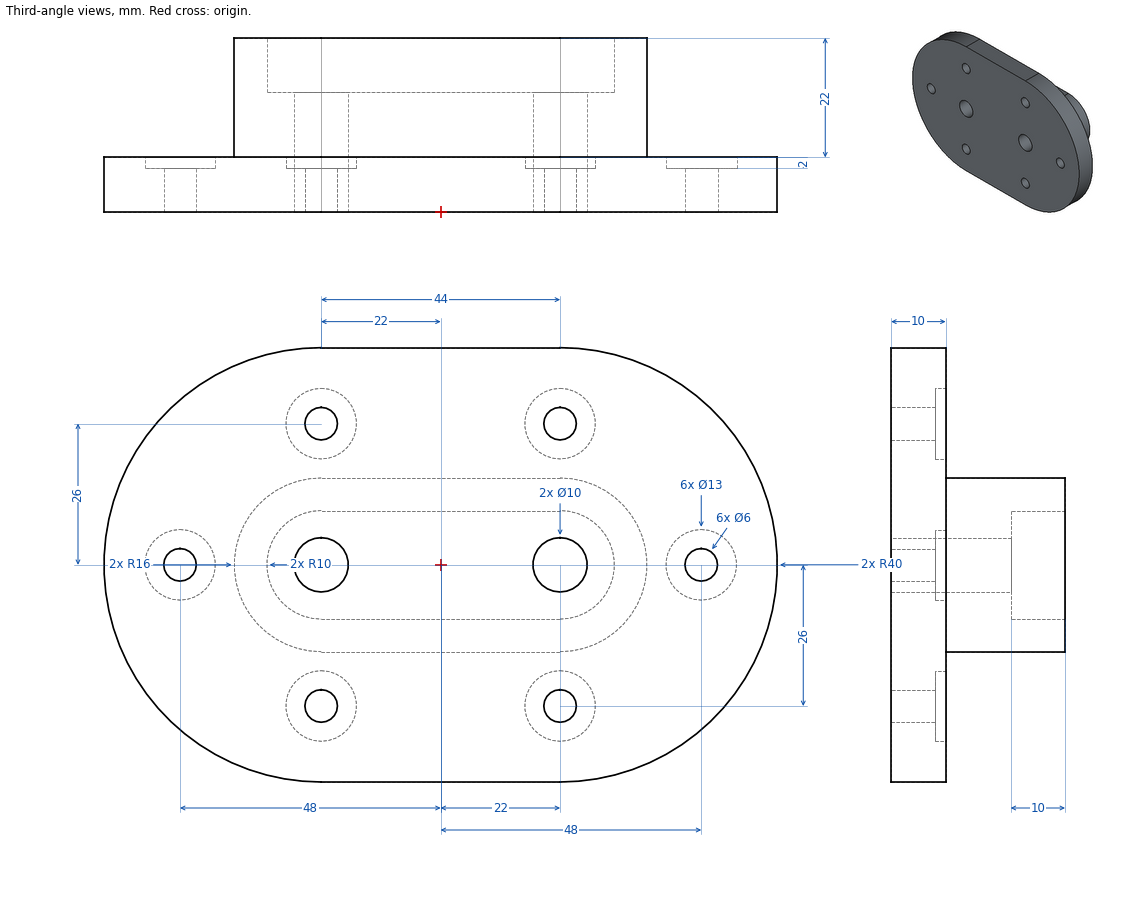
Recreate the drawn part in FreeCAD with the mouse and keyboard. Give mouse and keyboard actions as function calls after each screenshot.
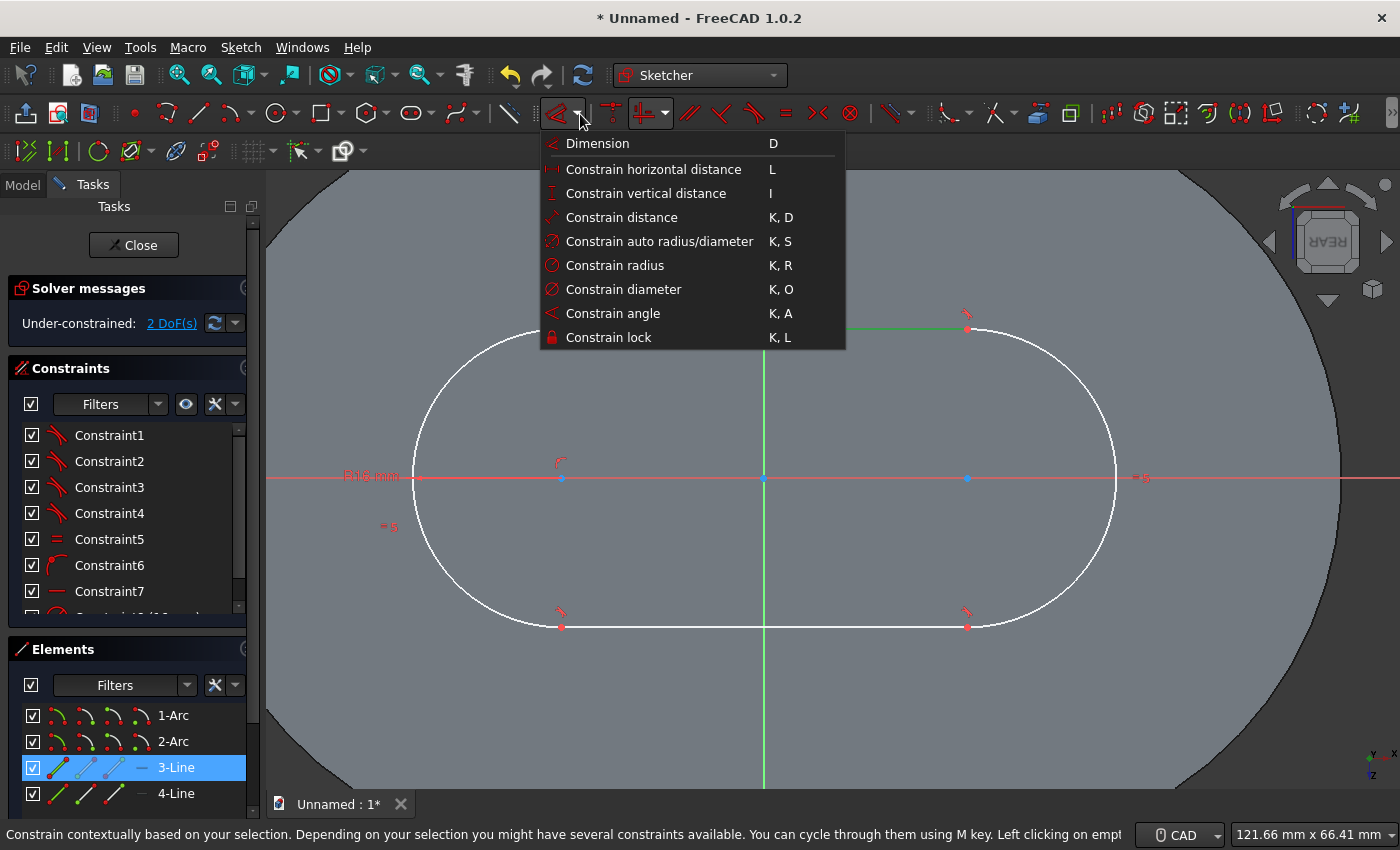
click(693, 169)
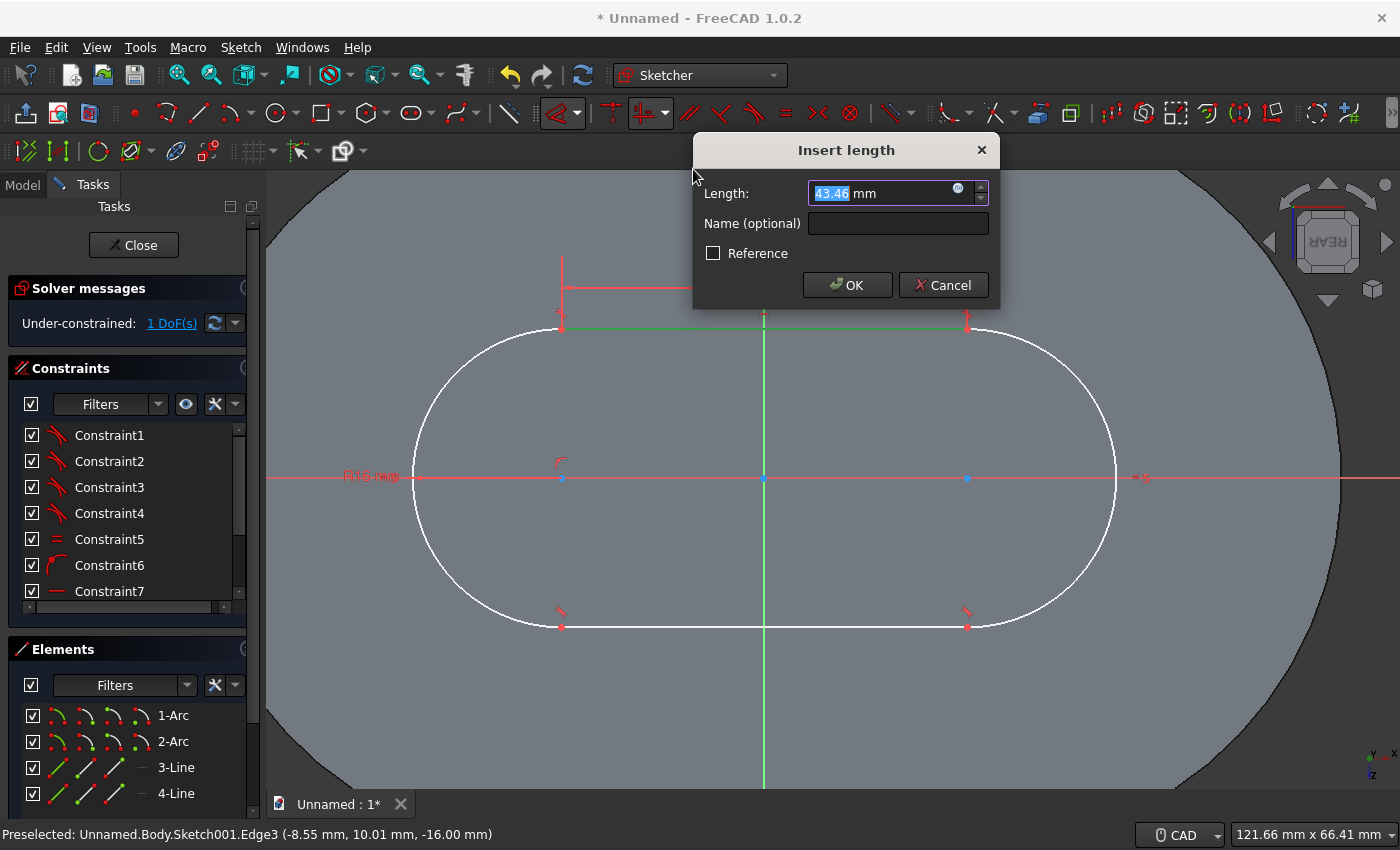
text(44)
key(Return)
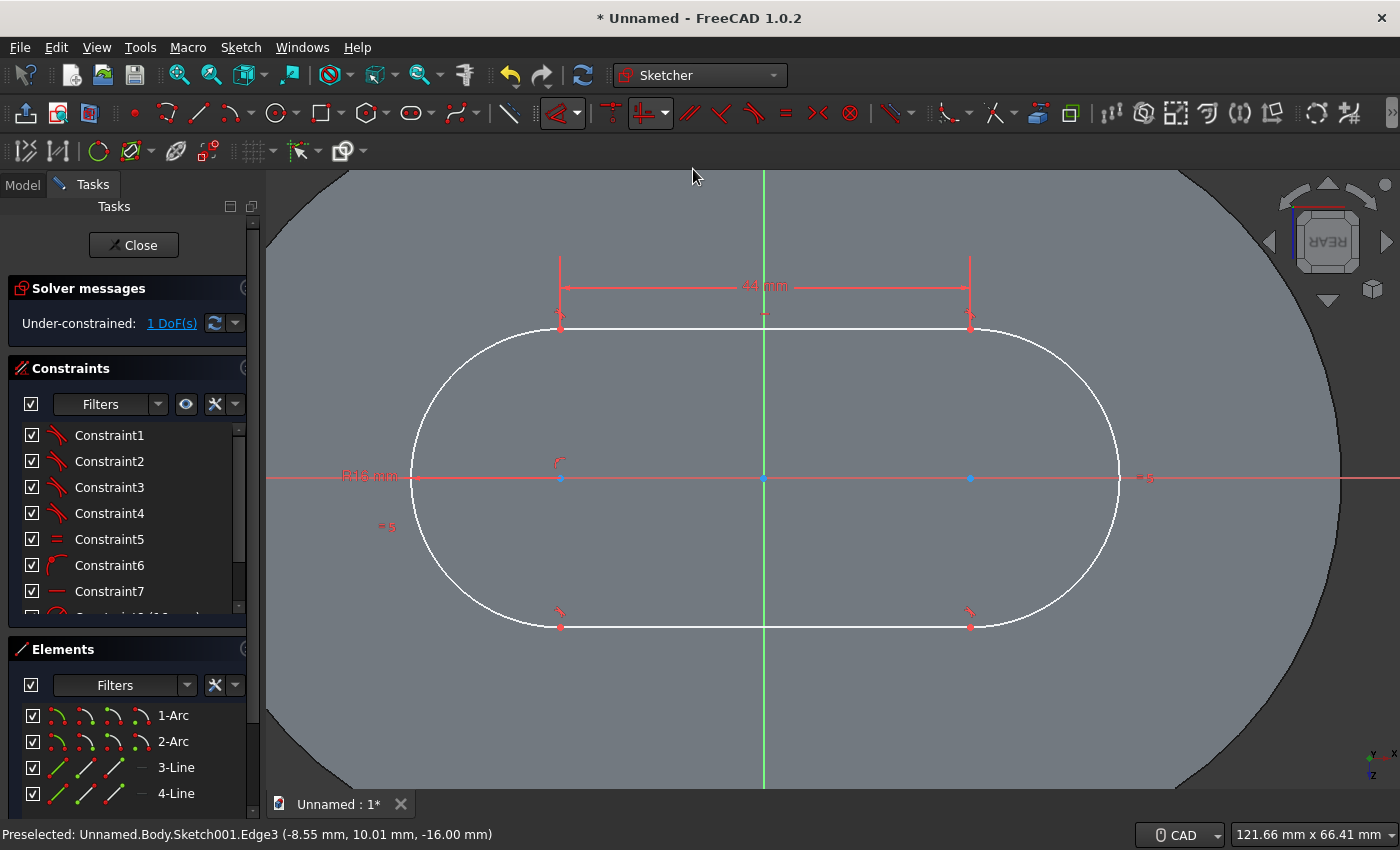
click(560, 329)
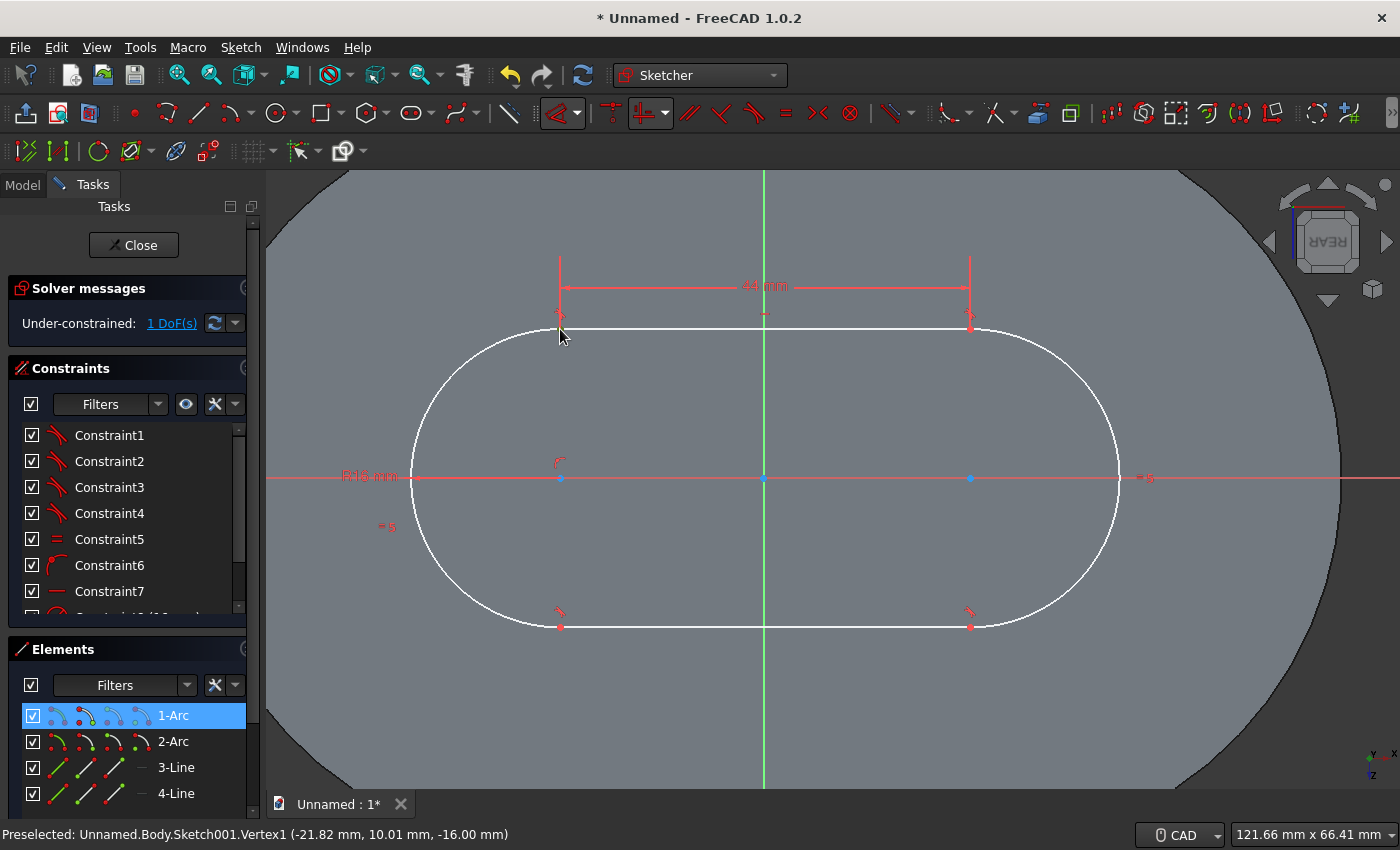
key(l)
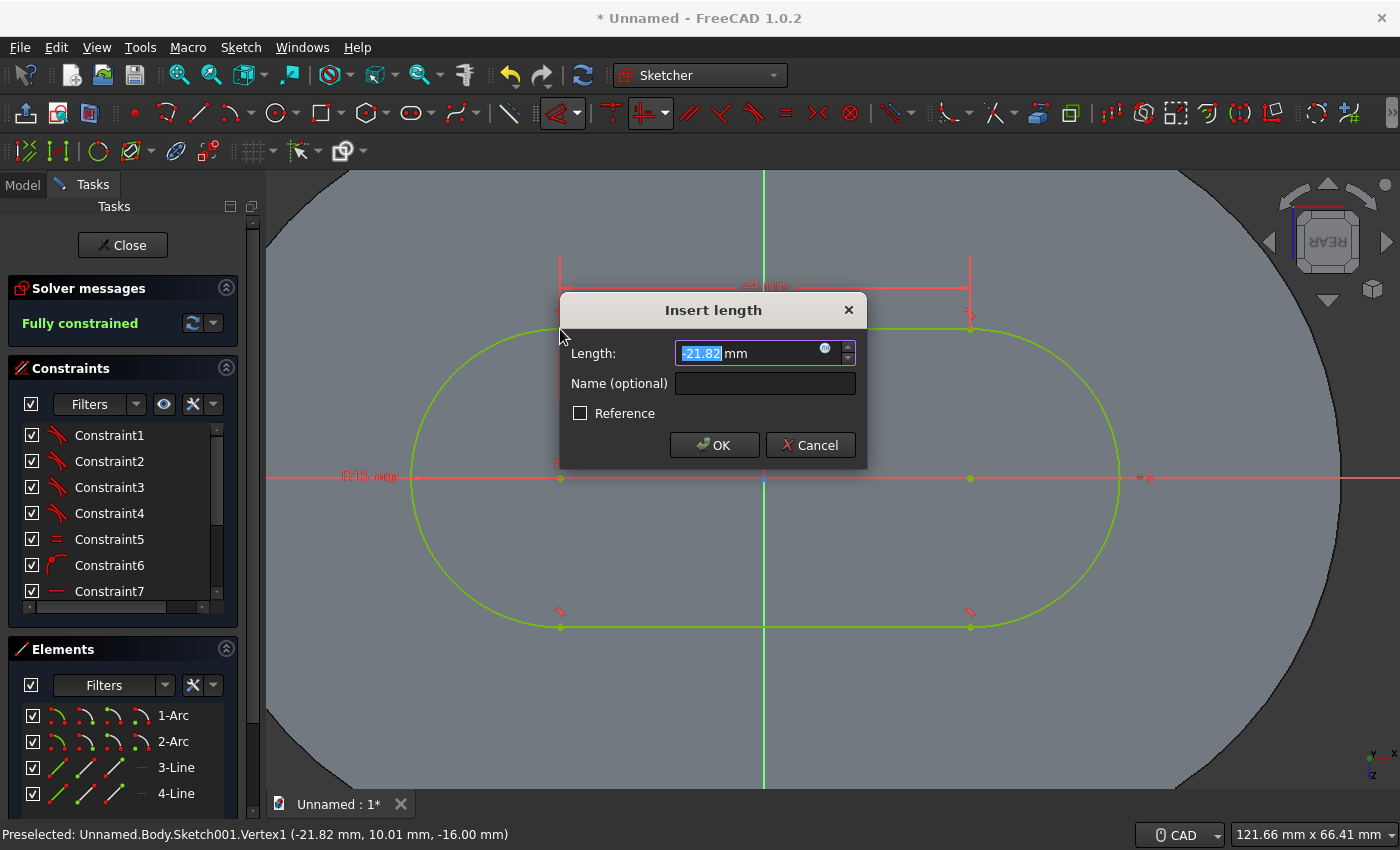
text(-22)
key(Return)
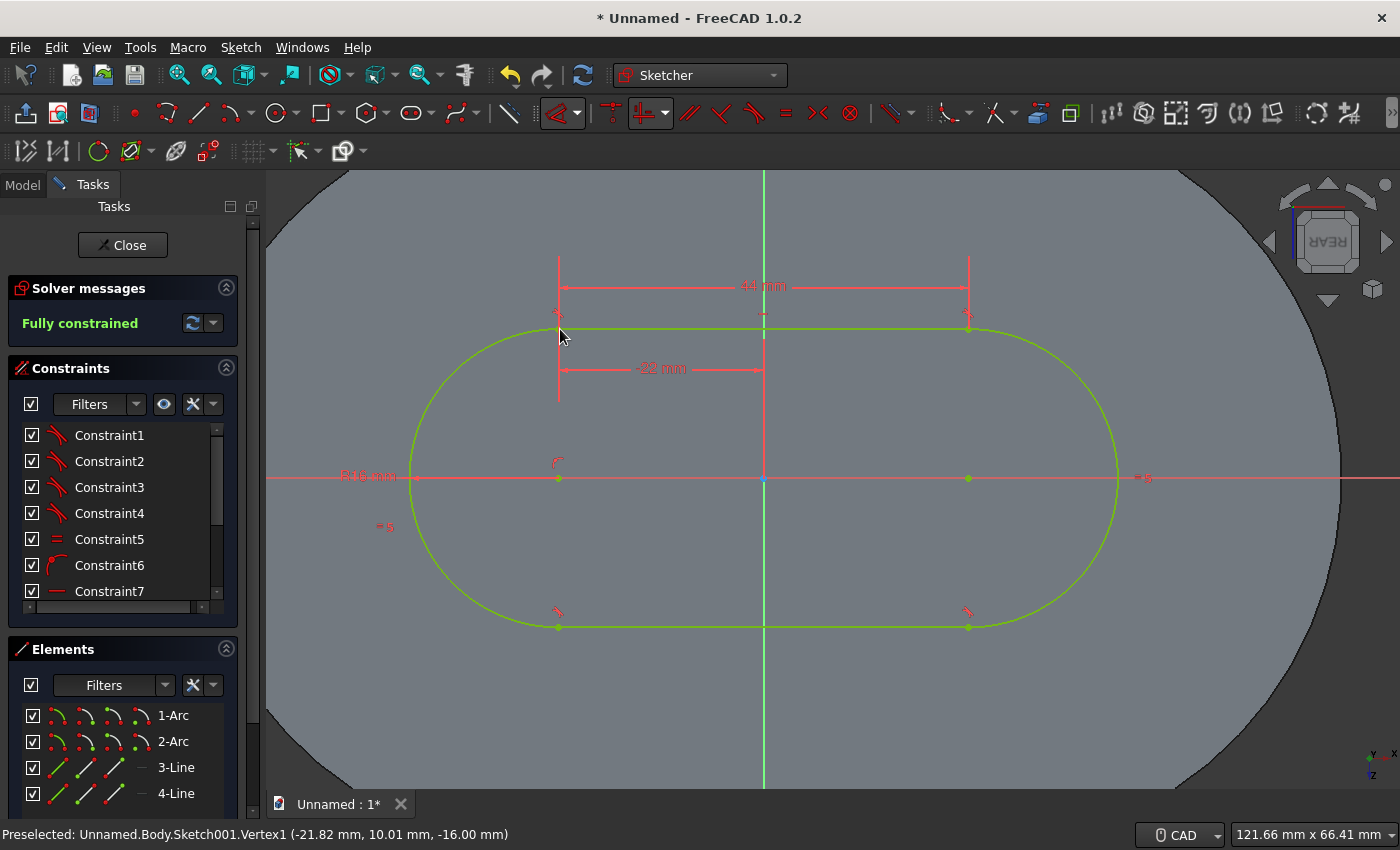
click(123, 245)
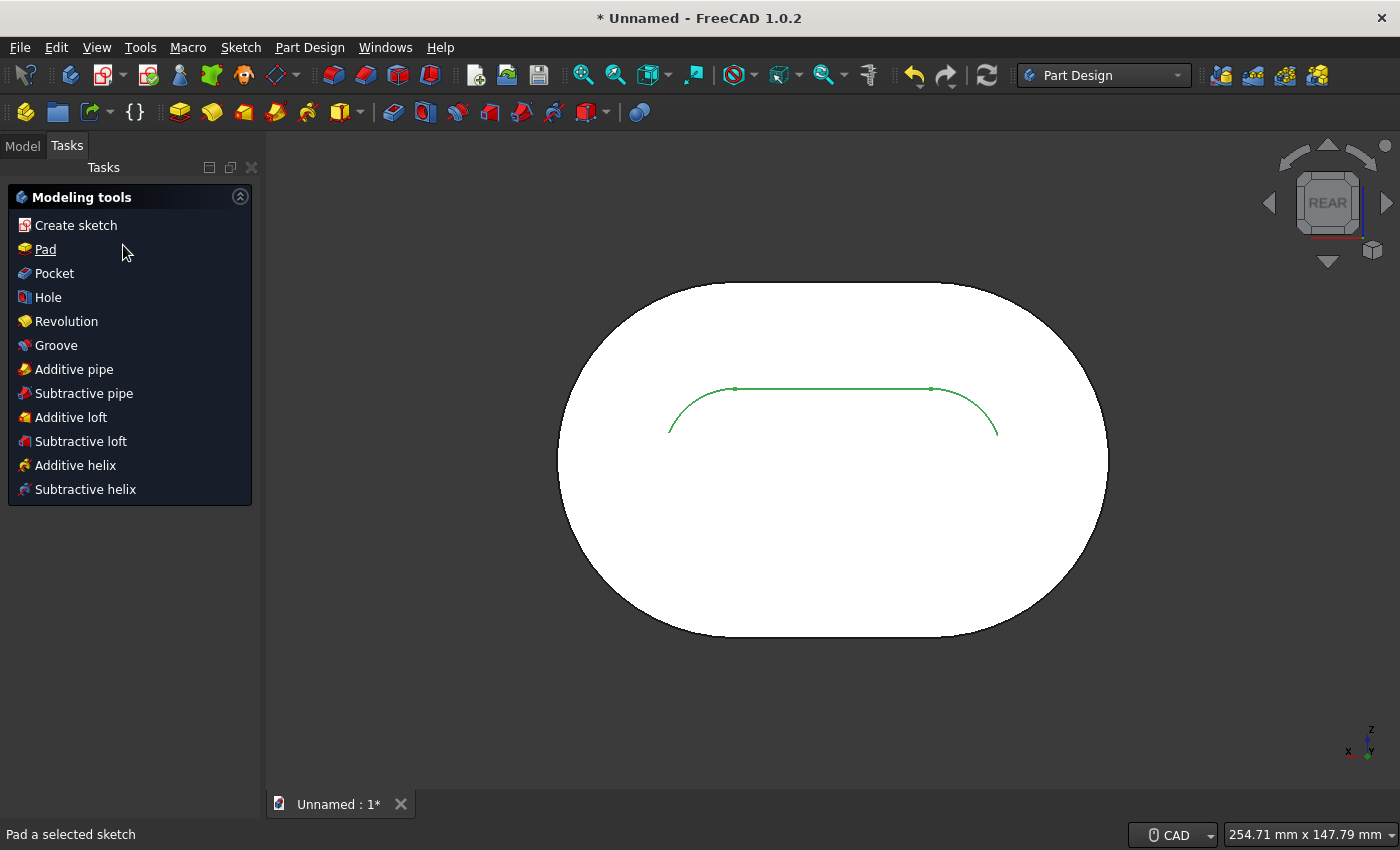
click(180, 112)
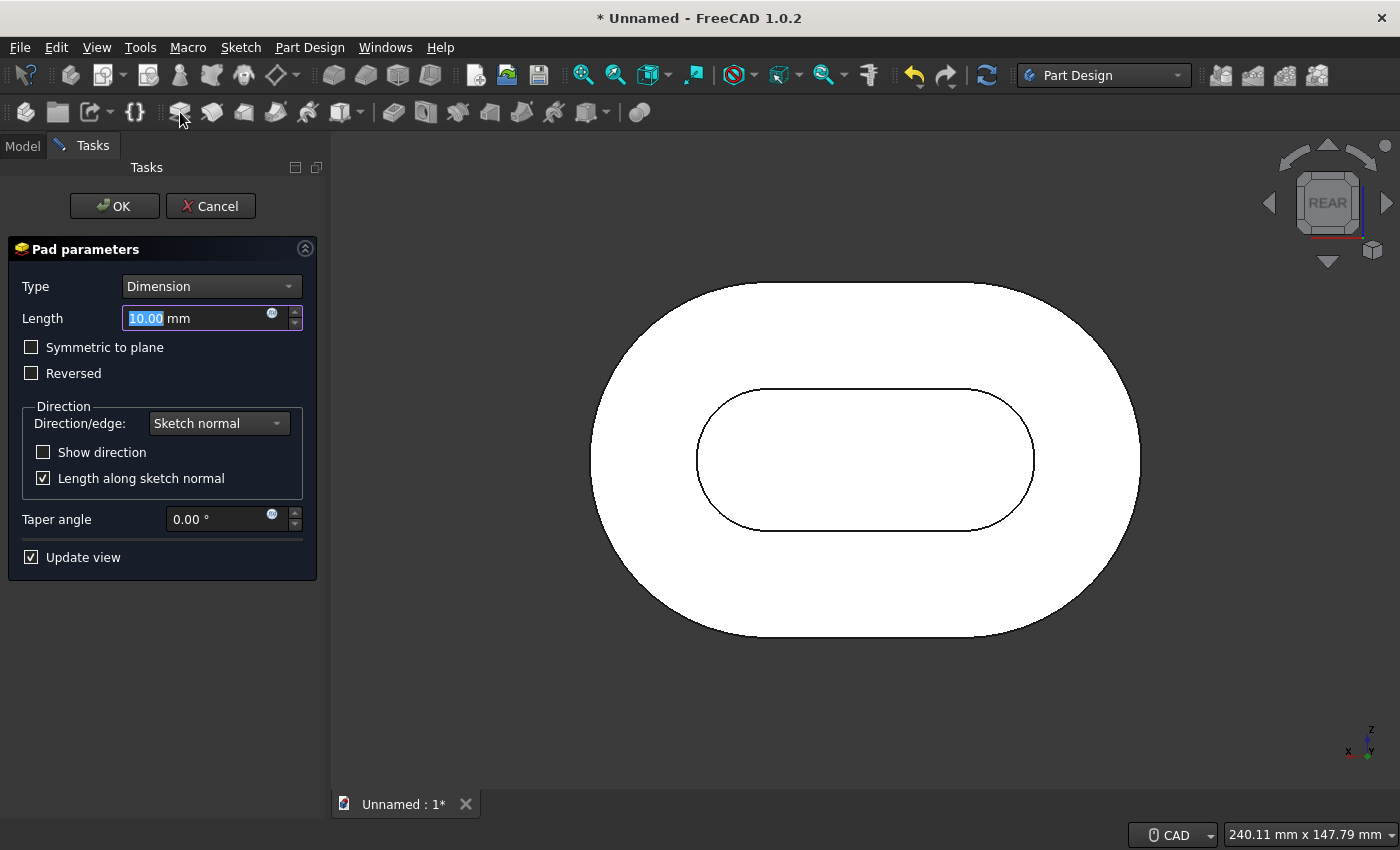
text(22)
key(Tab)